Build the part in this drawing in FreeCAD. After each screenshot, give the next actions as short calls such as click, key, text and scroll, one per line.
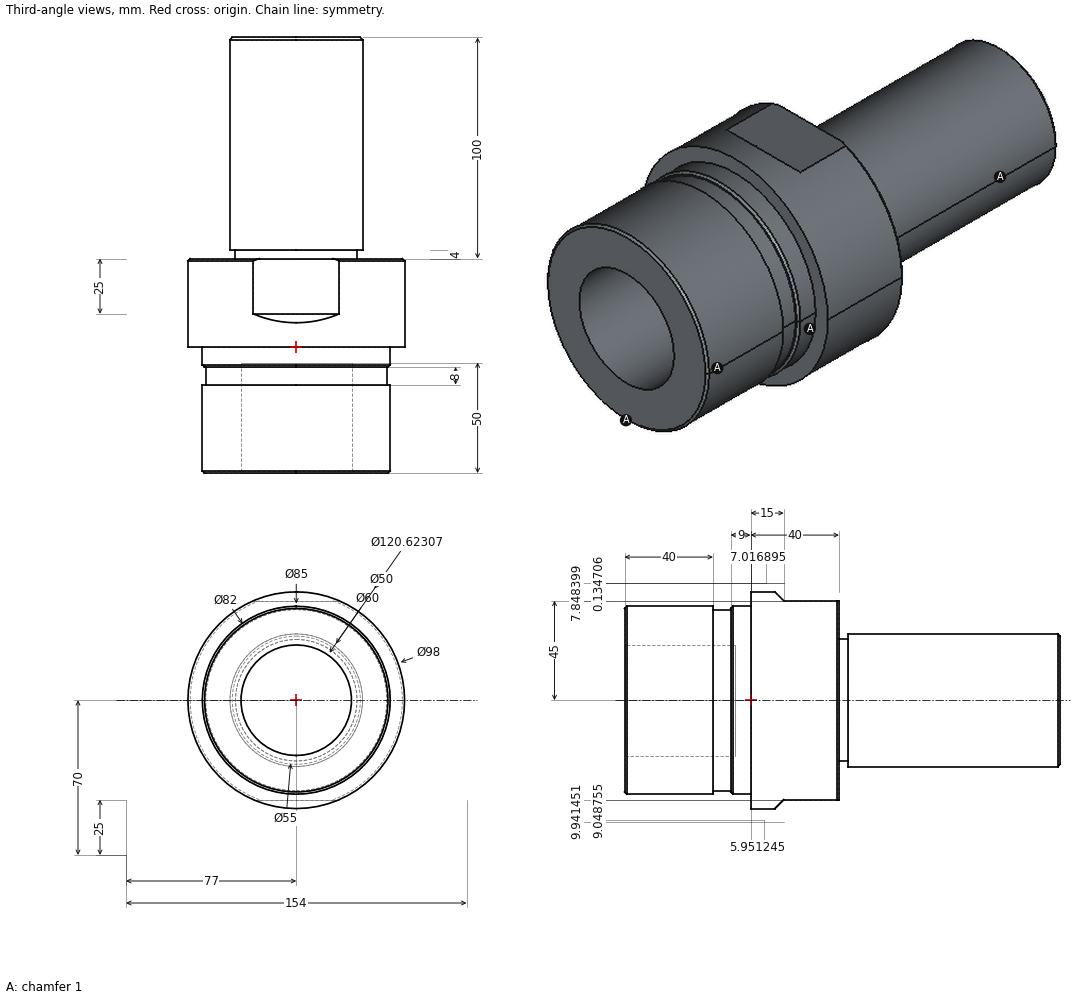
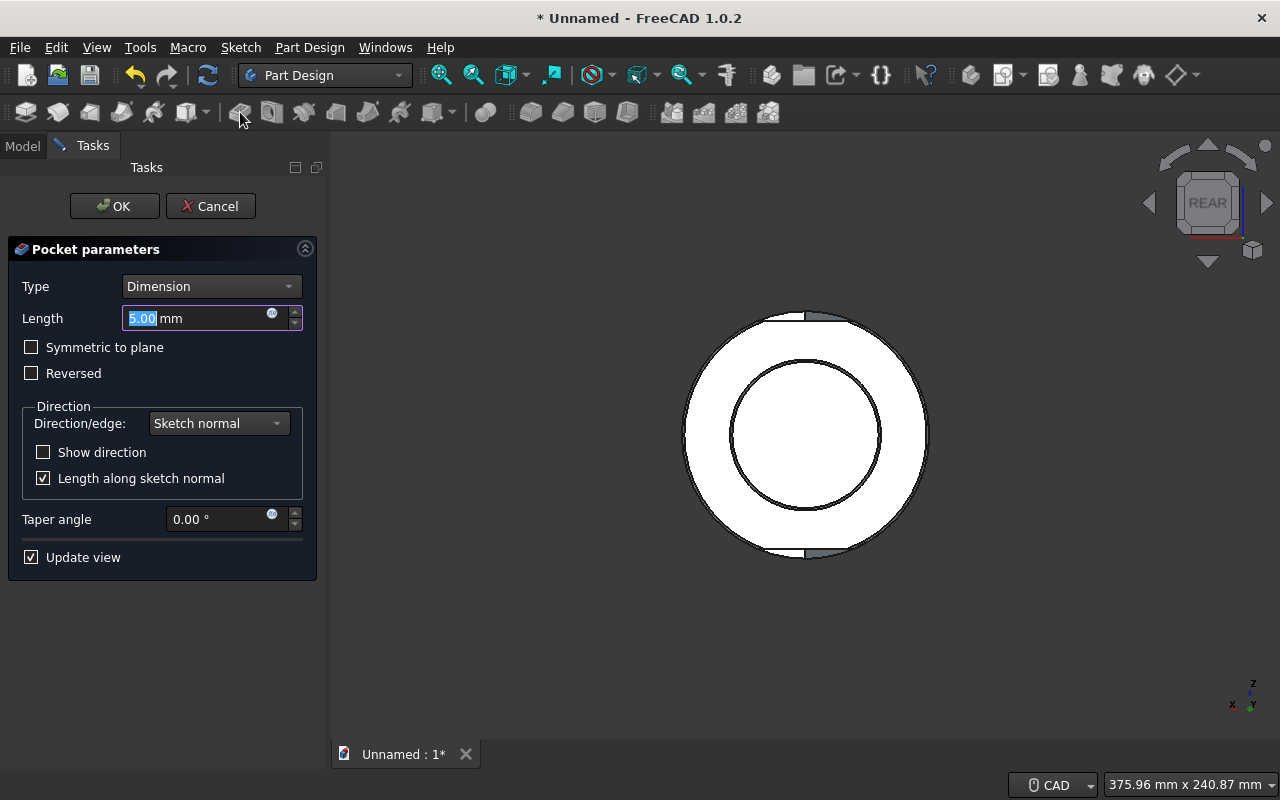
click(212, 286)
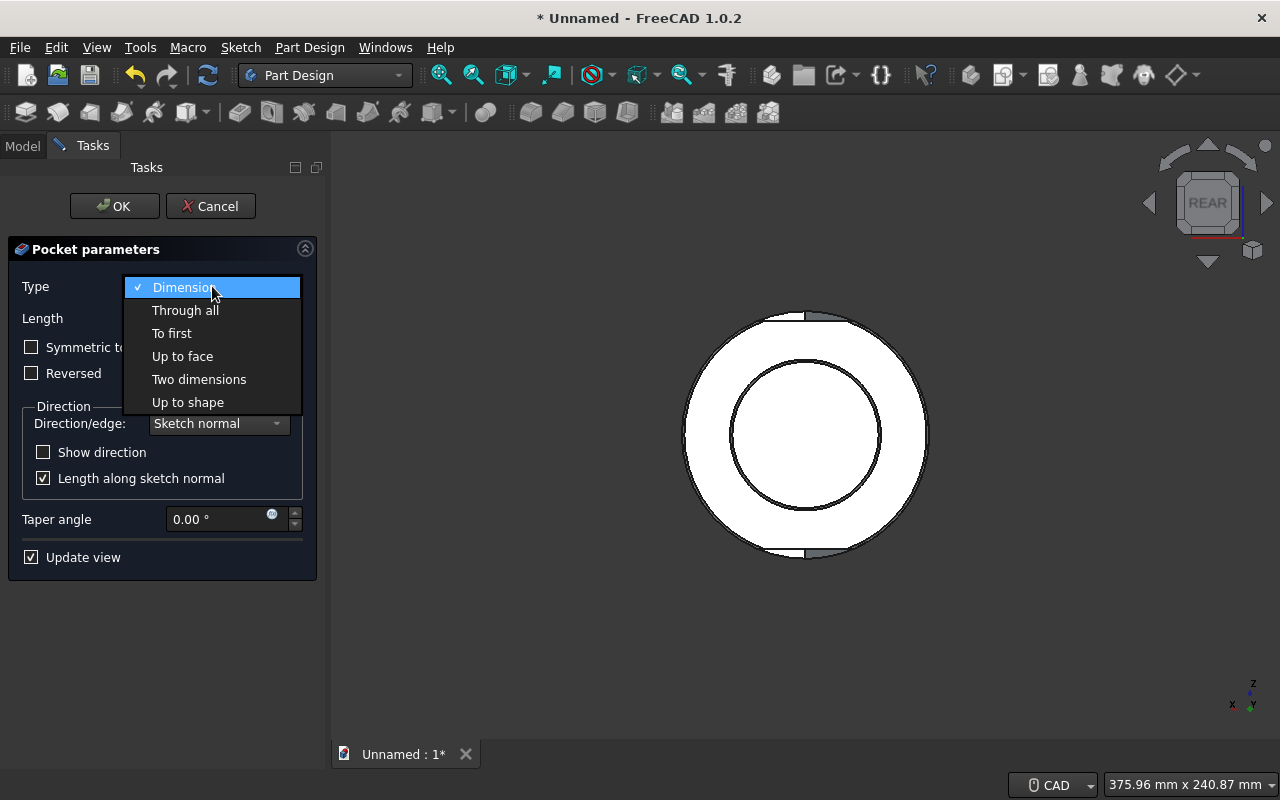
click(212, 310)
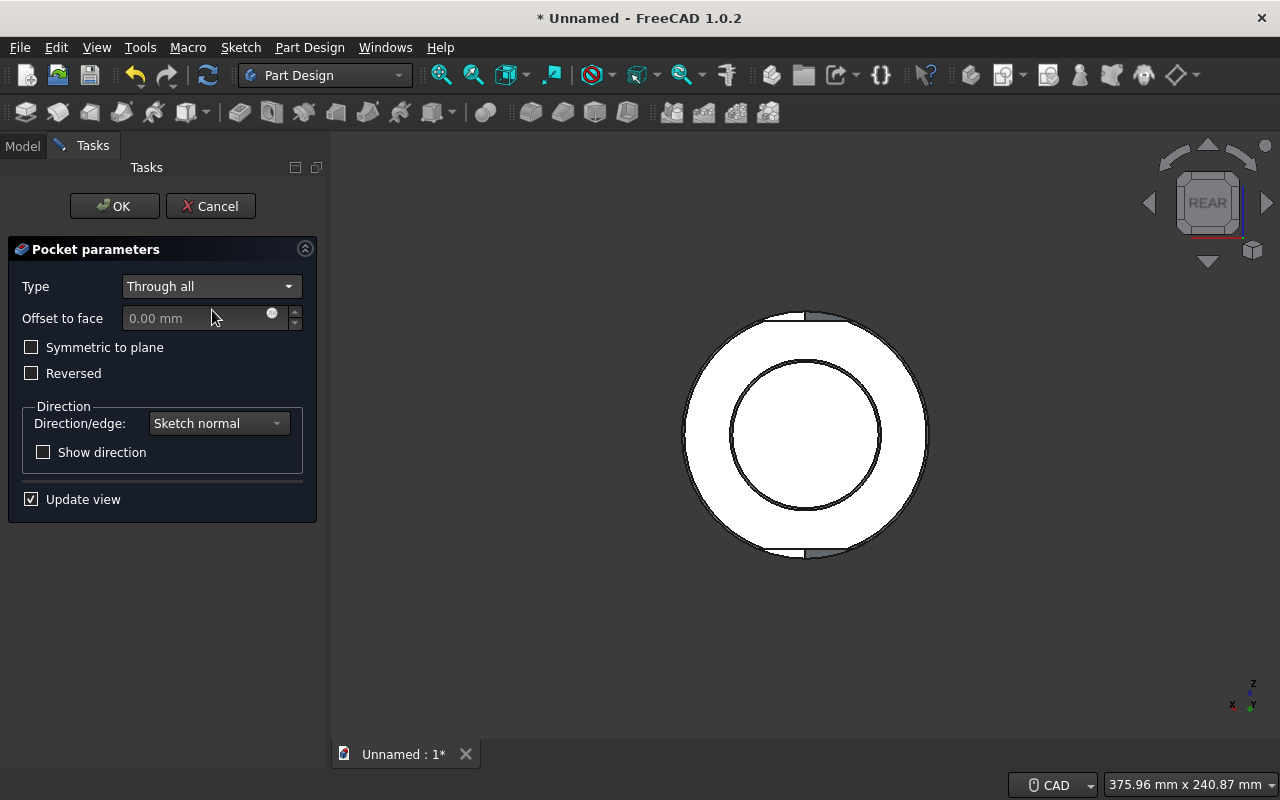
click(30, 373)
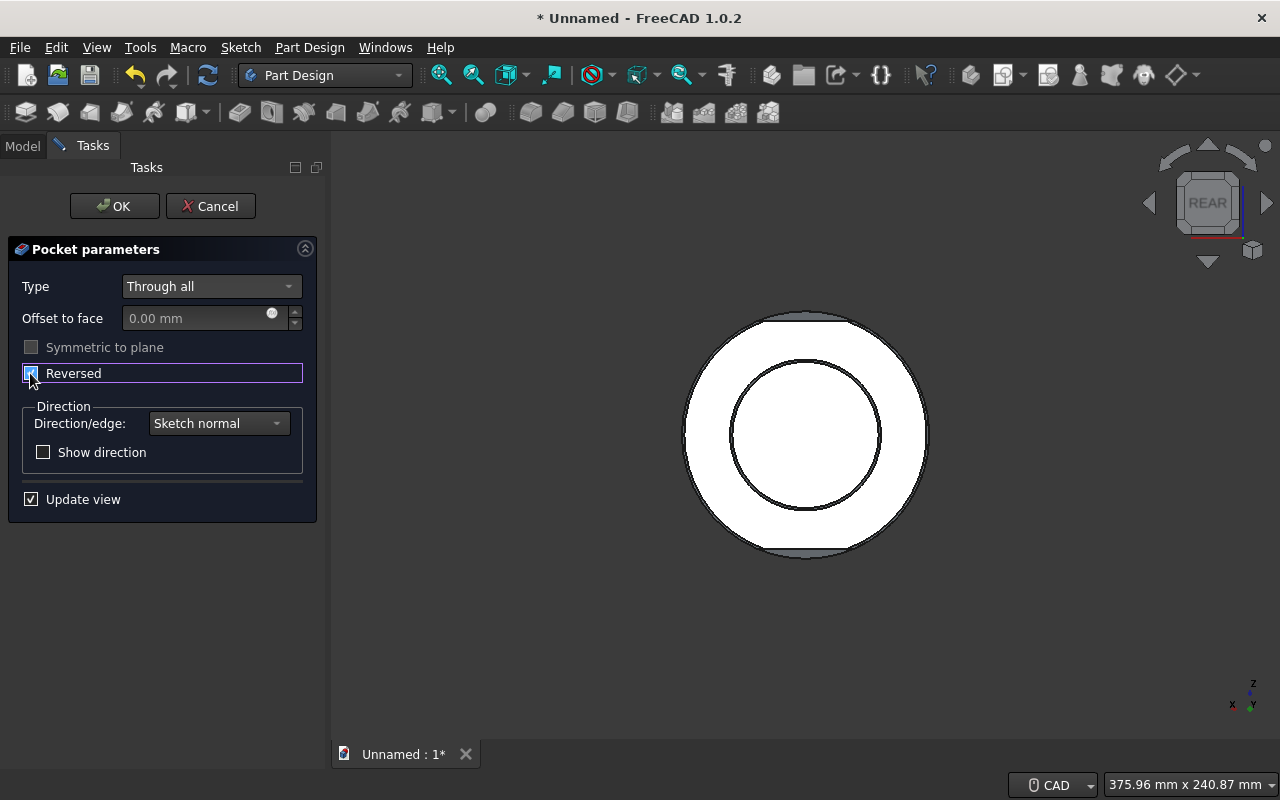
click(115, 206)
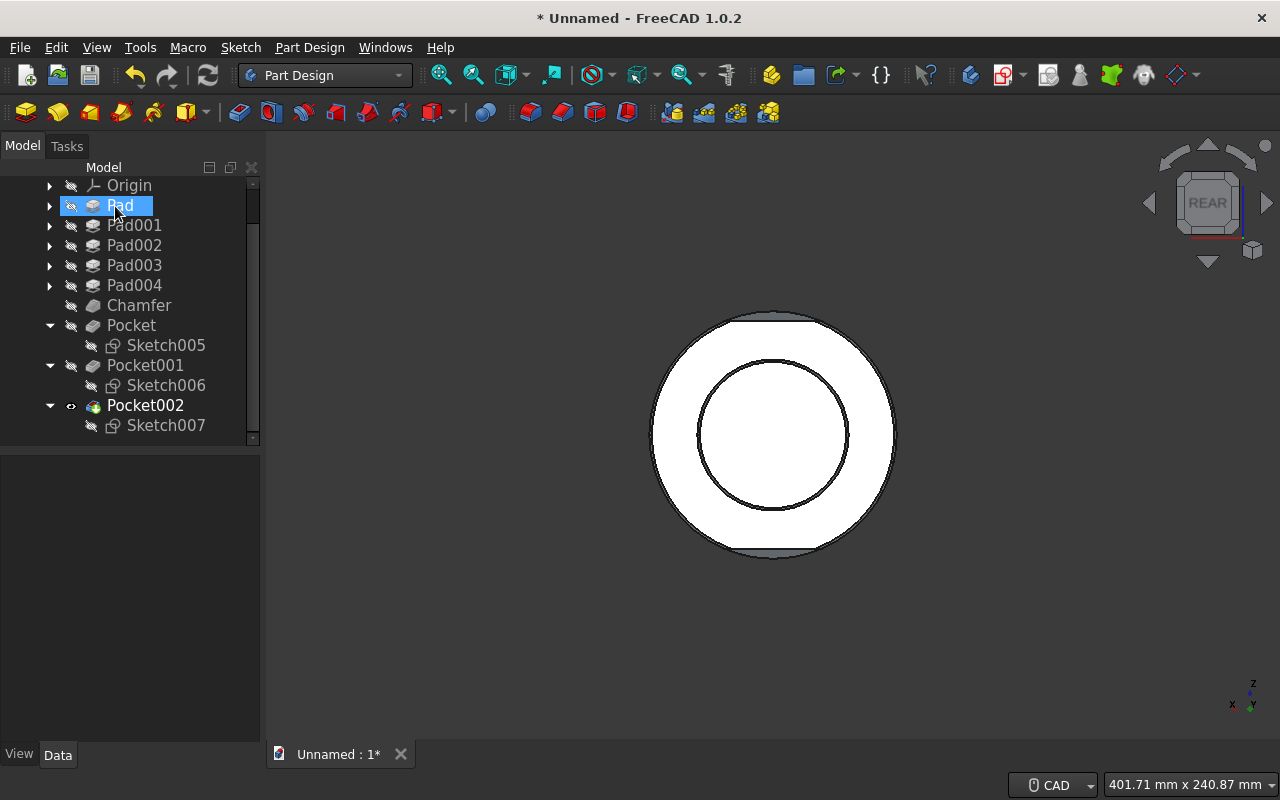
click(442, 76)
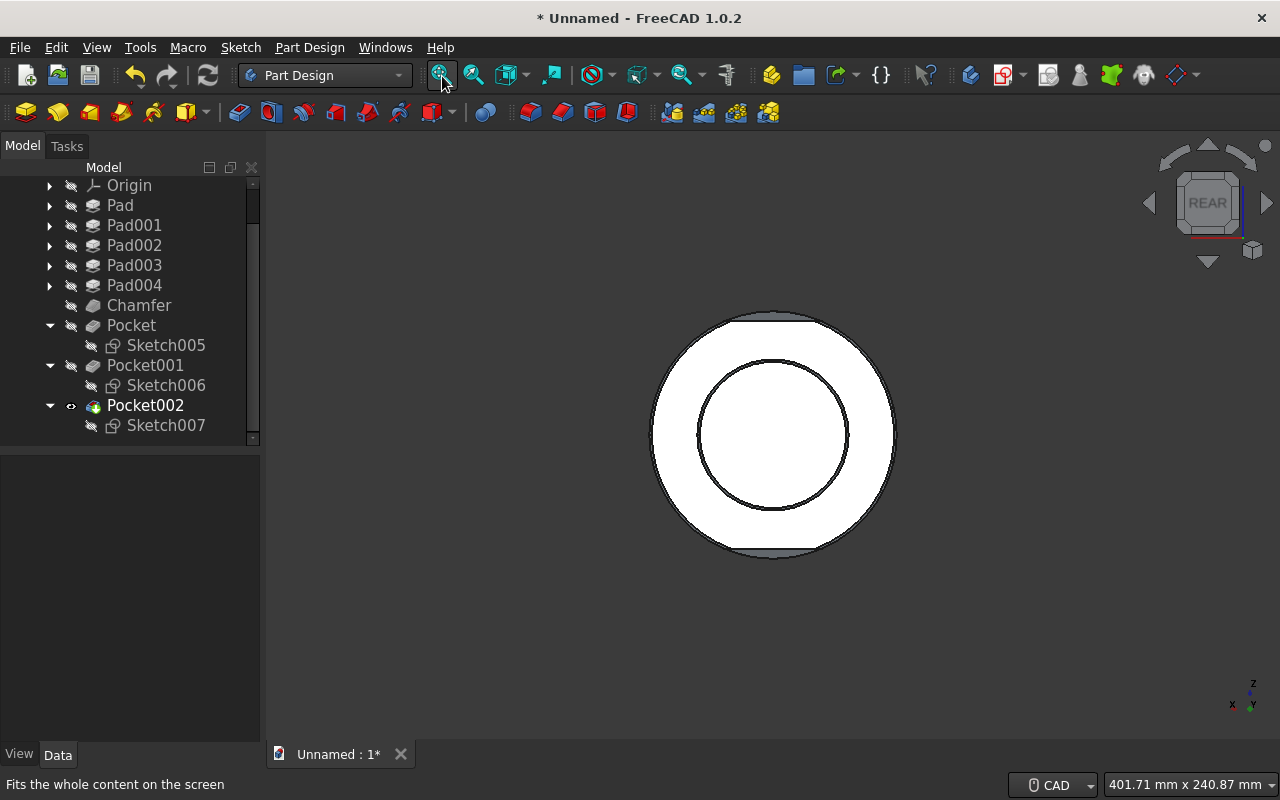
click(842, 499)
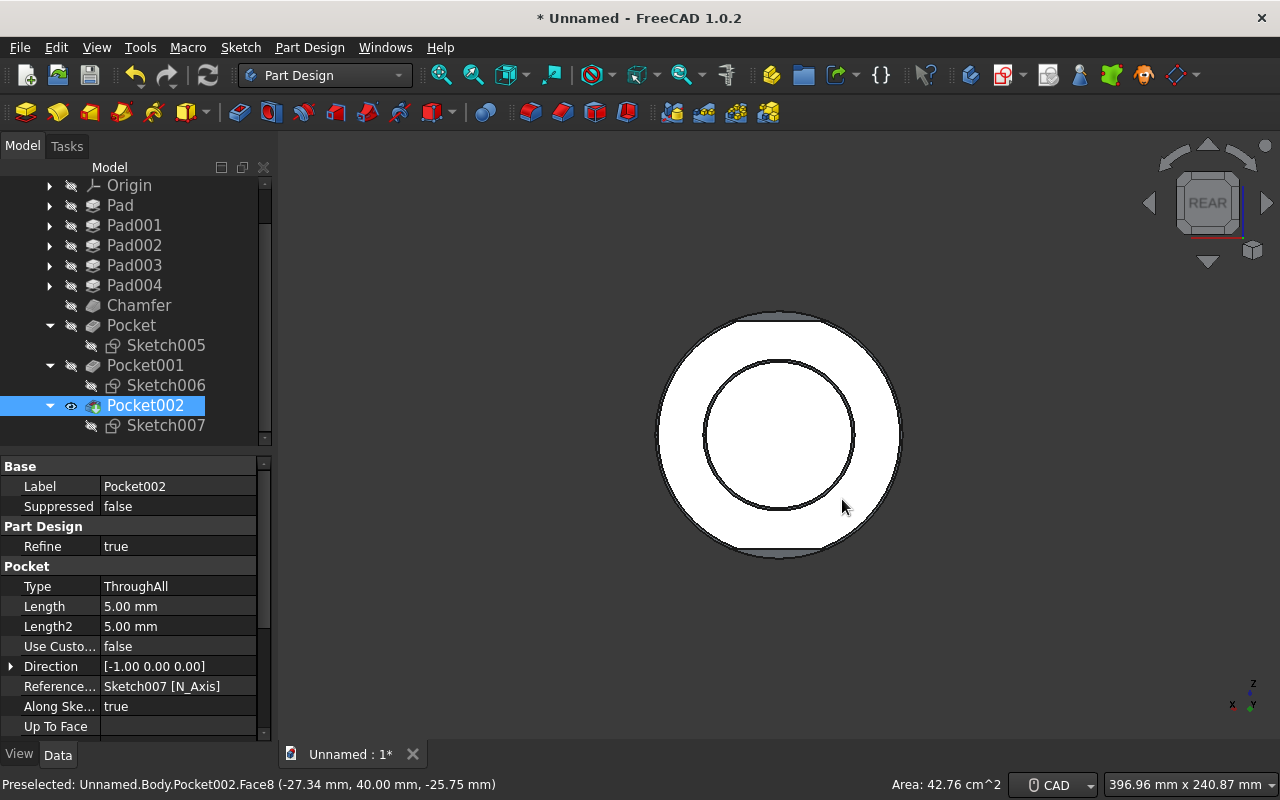
click(1004, 76)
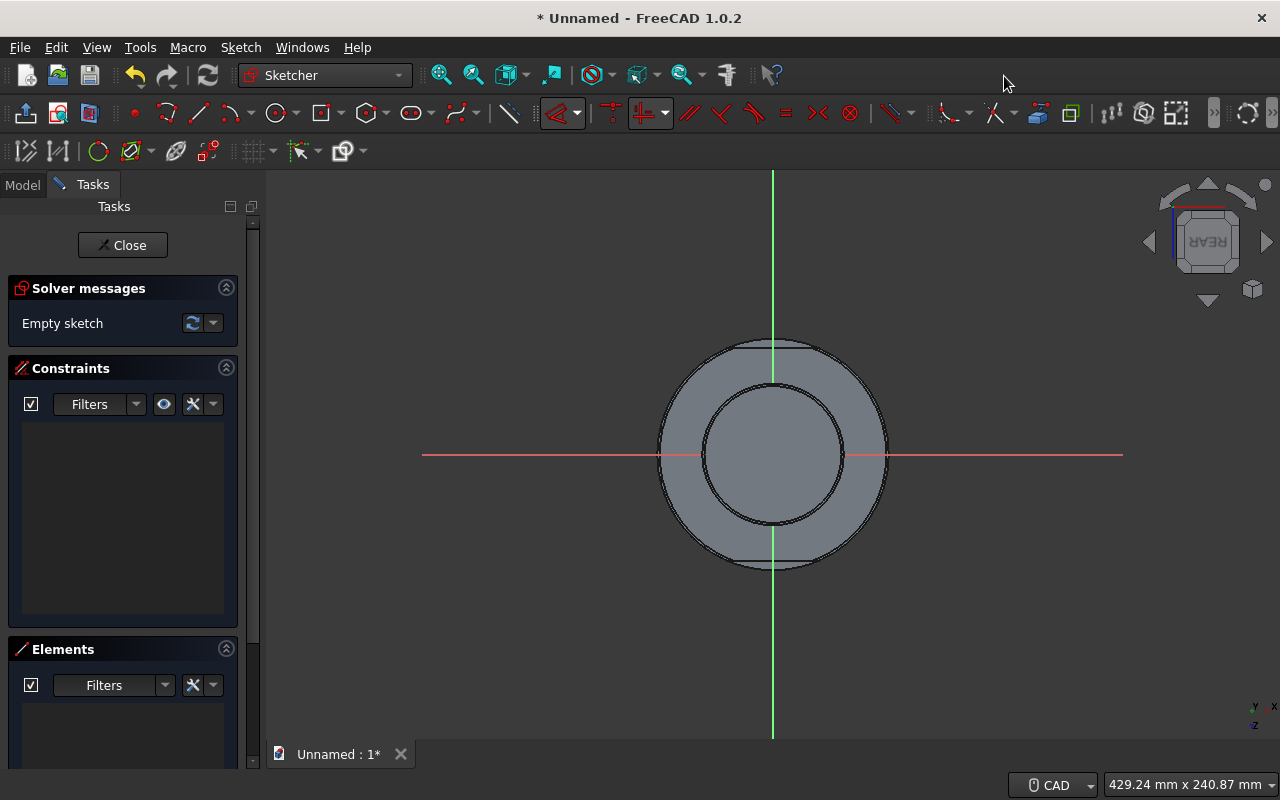
click(90, 114)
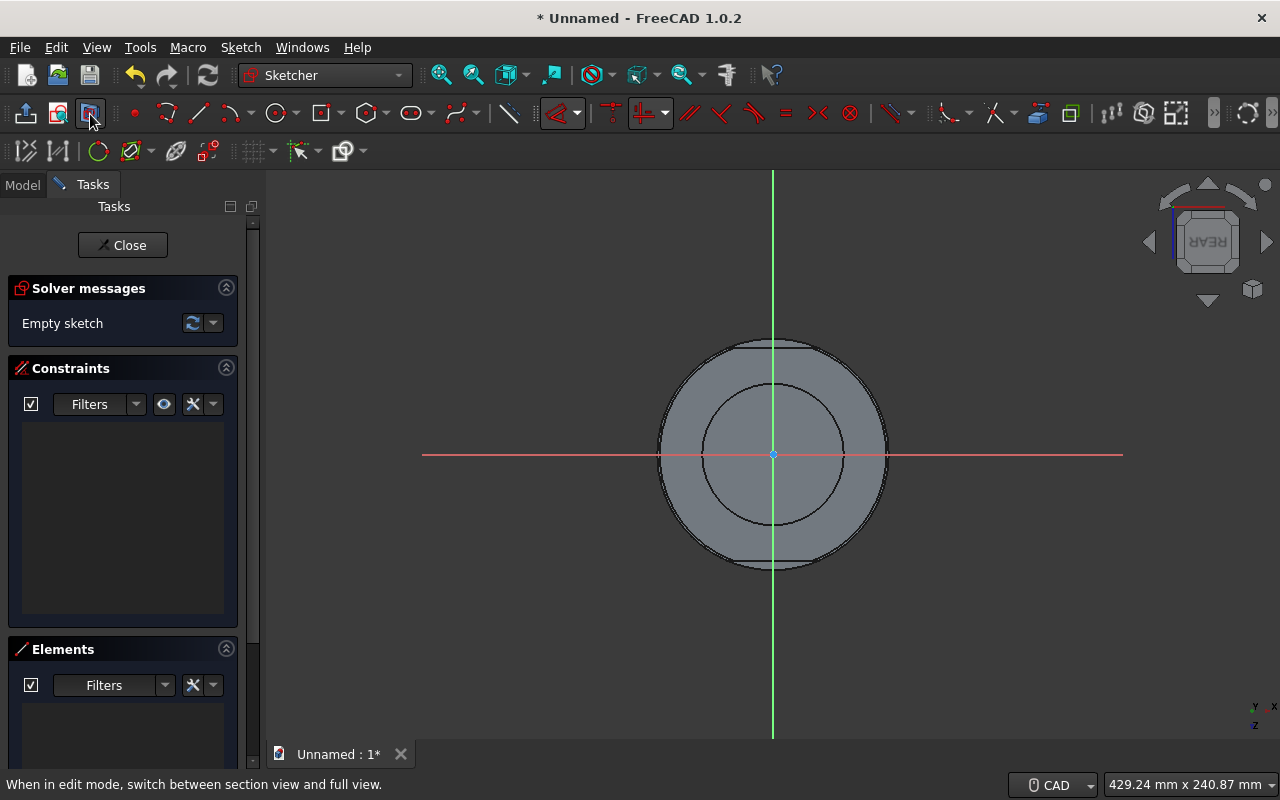
click(276, 114)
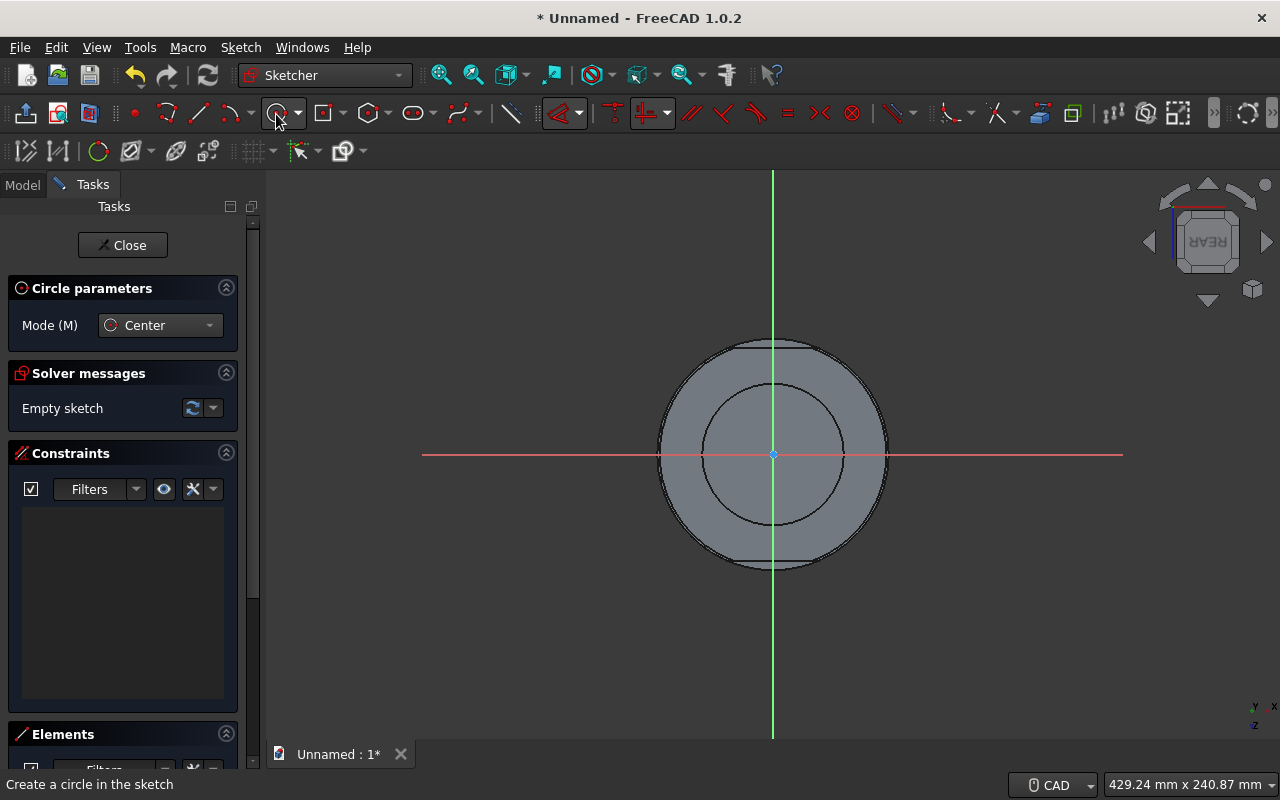
click(773, 454)
click(874, 354)